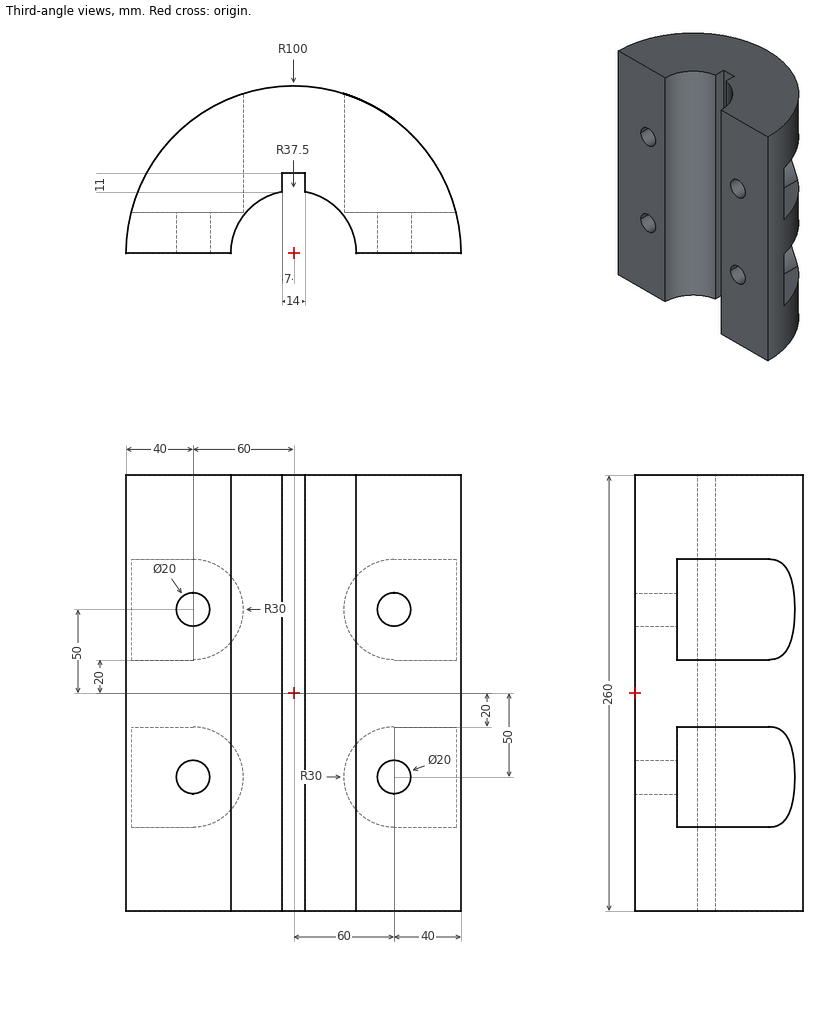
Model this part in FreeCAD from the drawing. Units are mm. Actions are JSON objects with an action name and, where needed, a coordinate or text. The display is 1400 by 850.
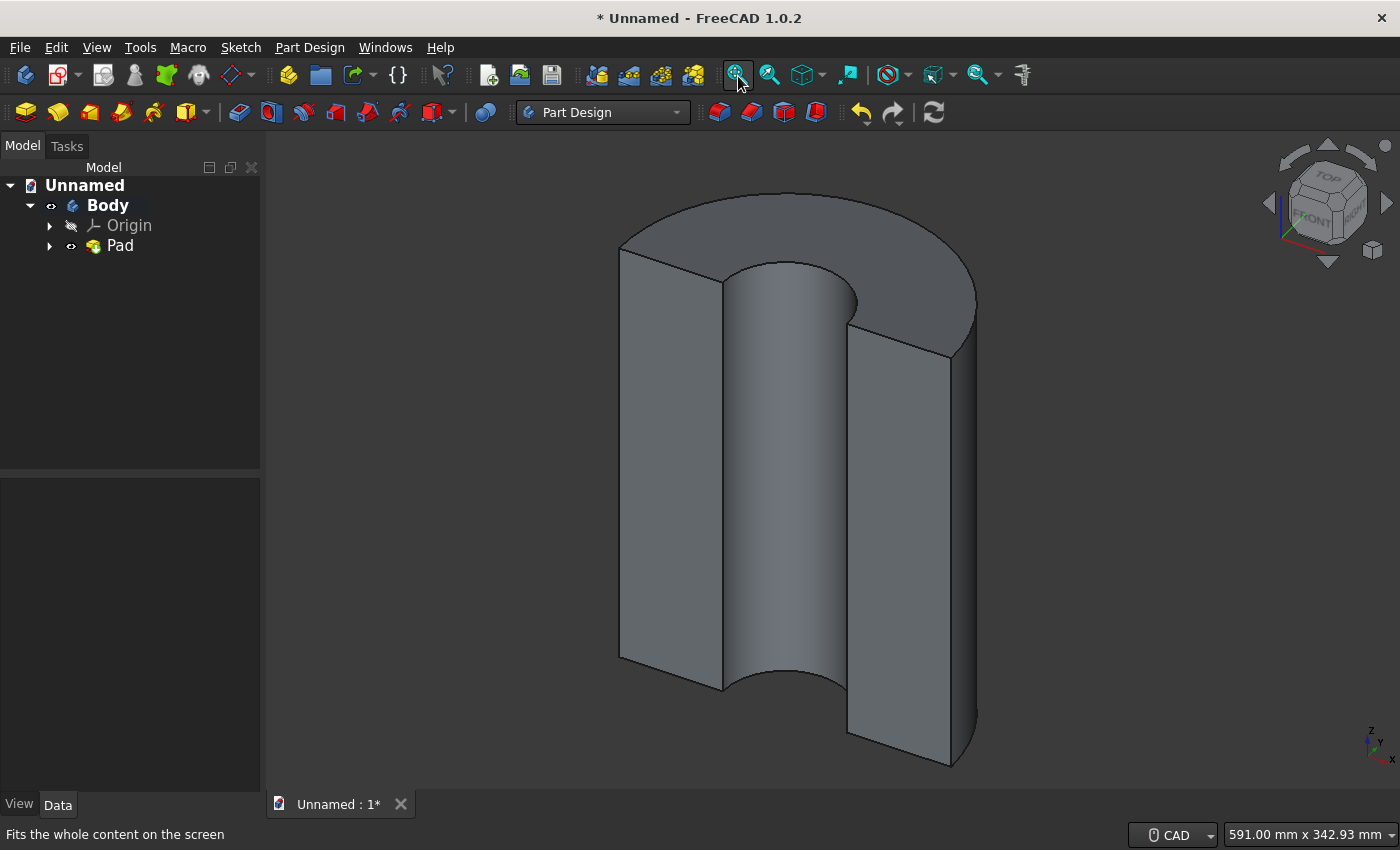
{"action": "left_click", "coordinate": [50, 226]}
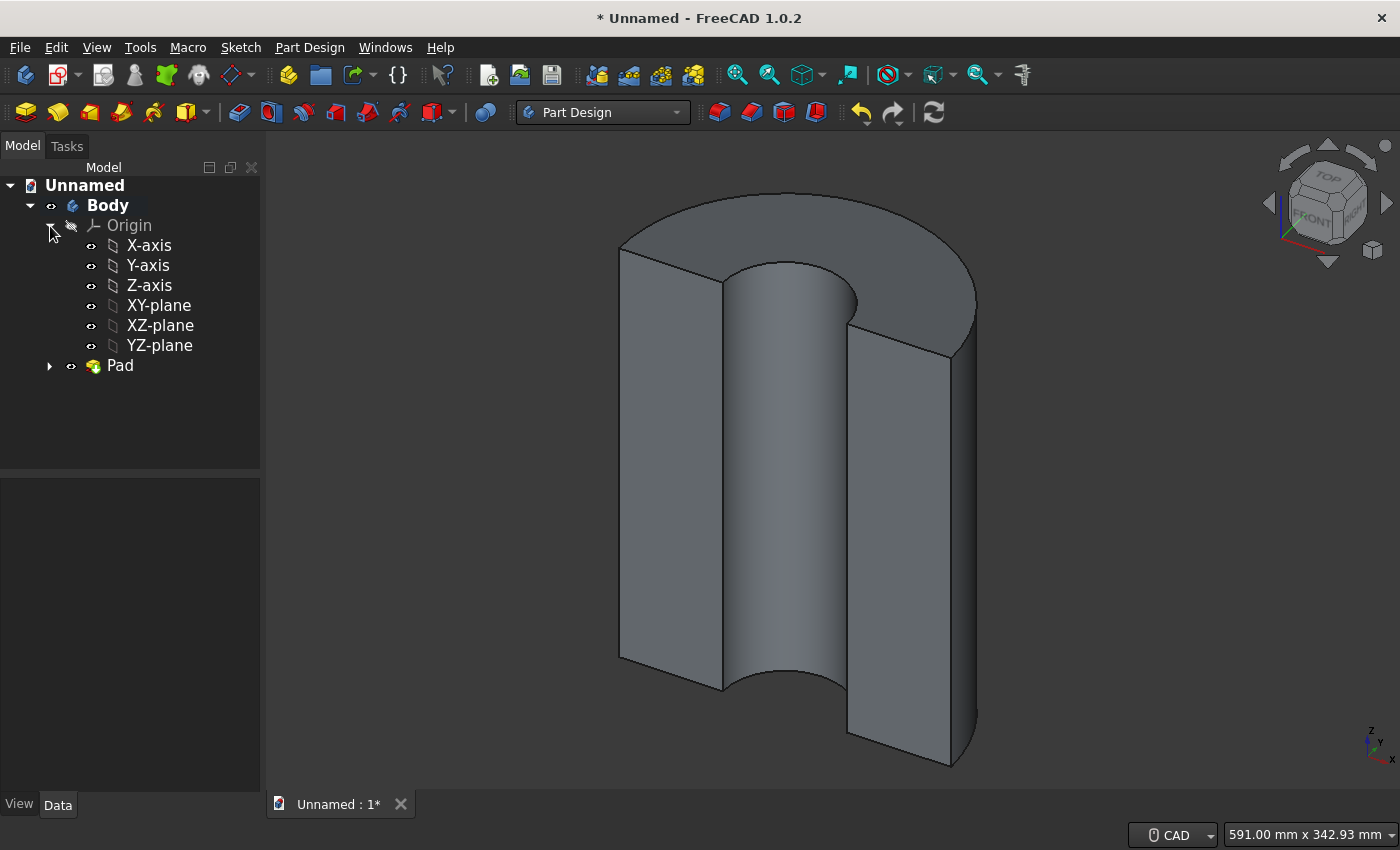
{"action": "left_click", "coordinate": [136, 326]}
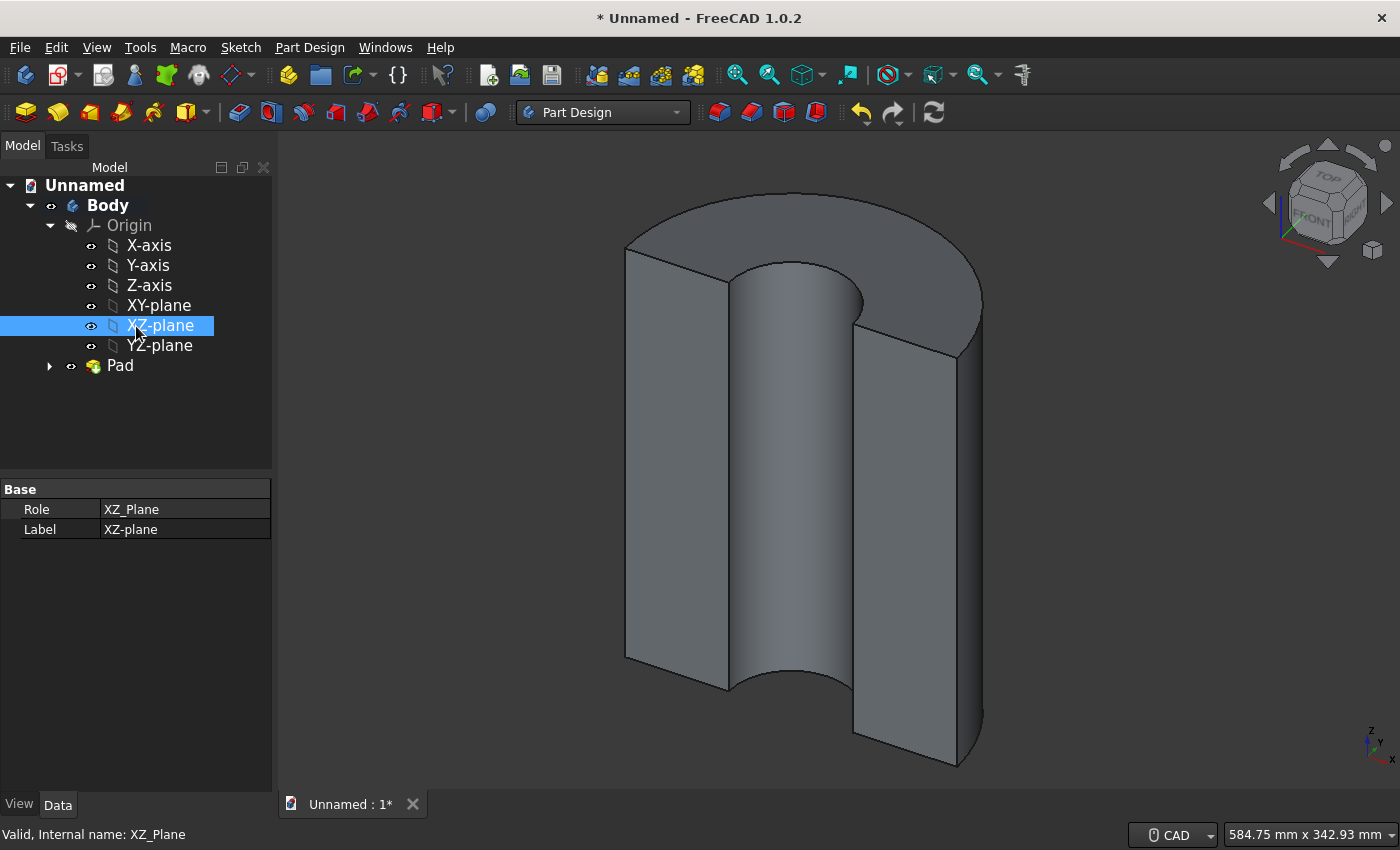
{"action": "left_click", "coordinate": [232, 76]}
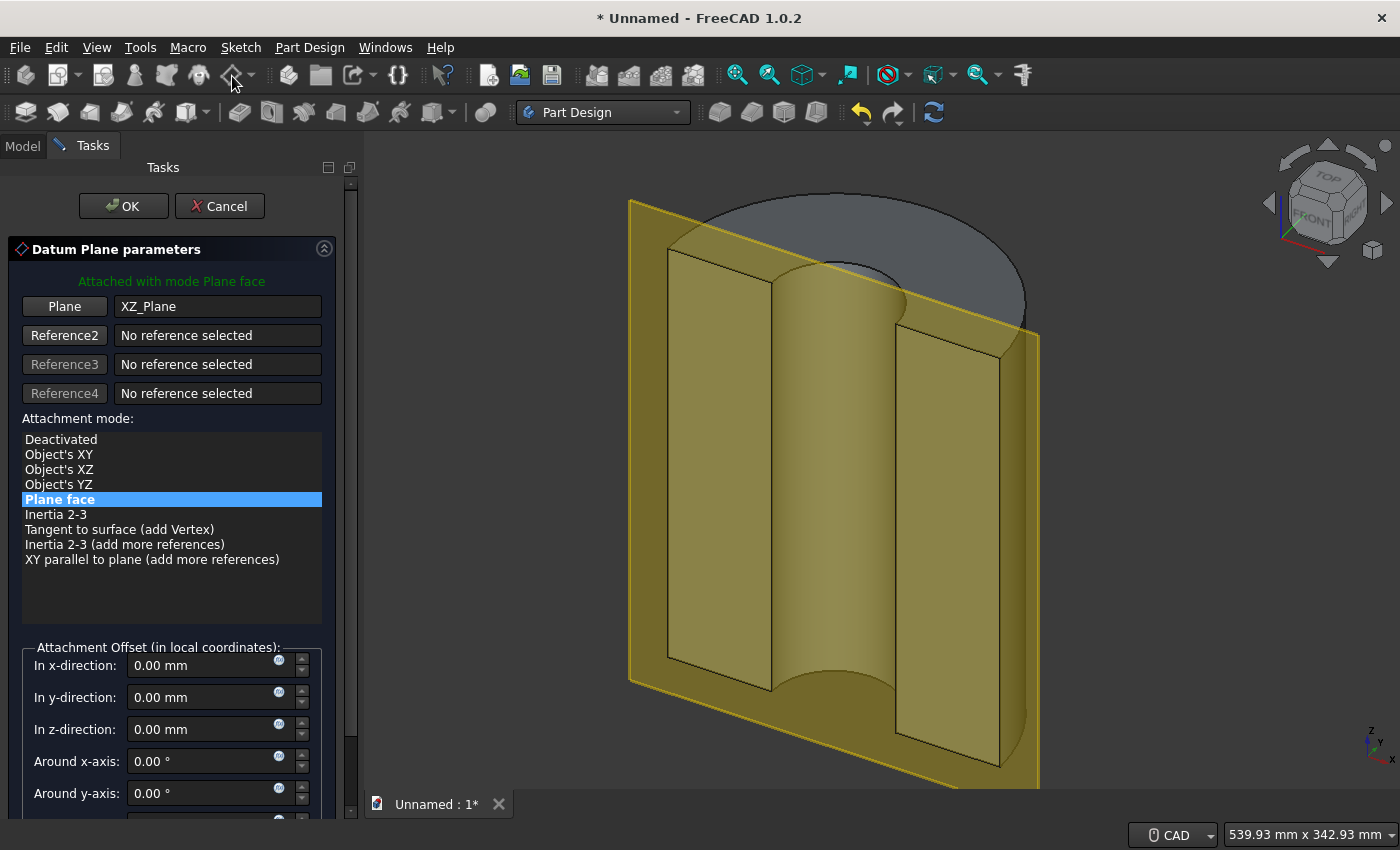
{"action": "triple_click", "coordinate": [210, 729]}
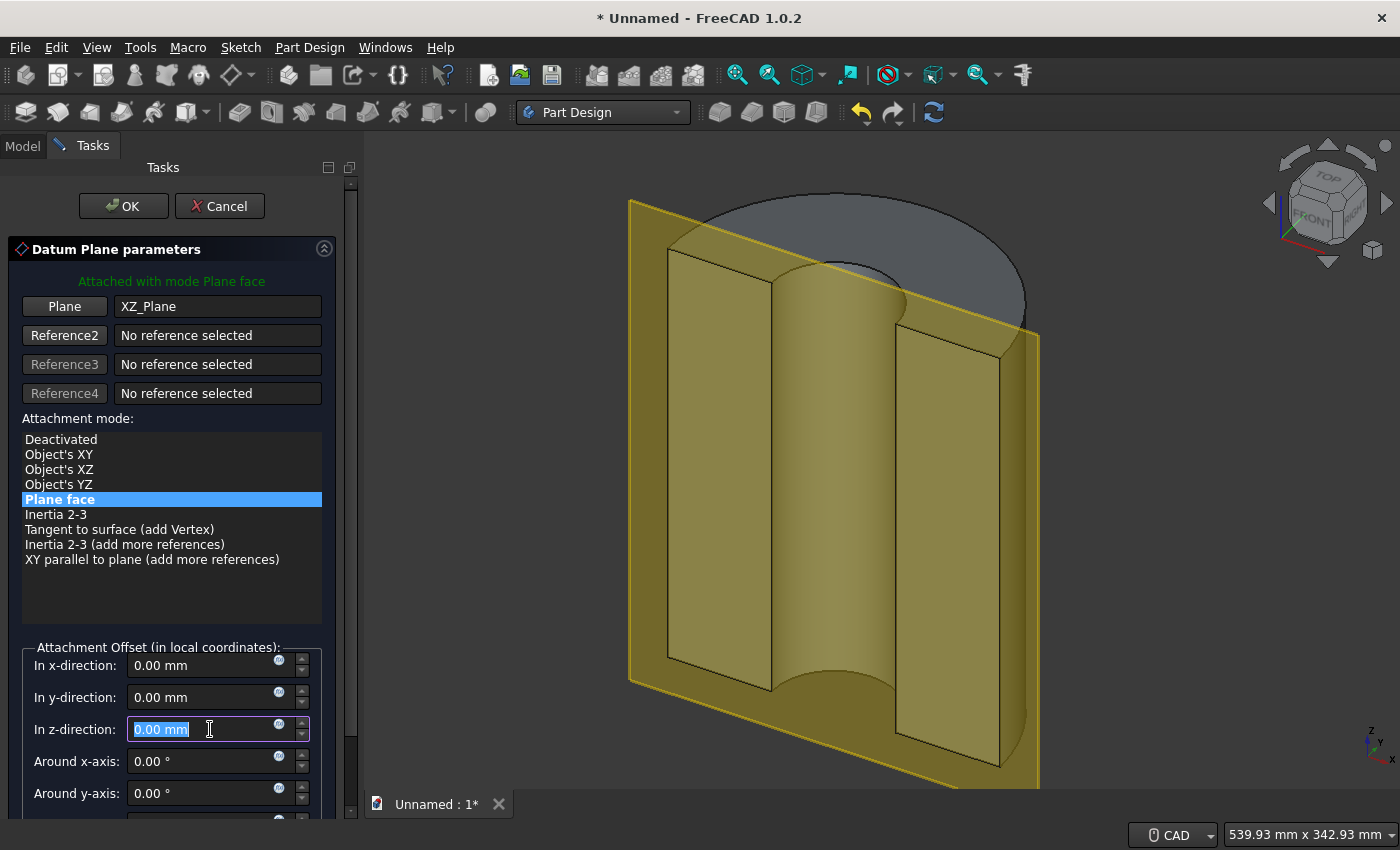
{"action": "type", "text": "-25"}
{"action": "key", "text": "Tab"}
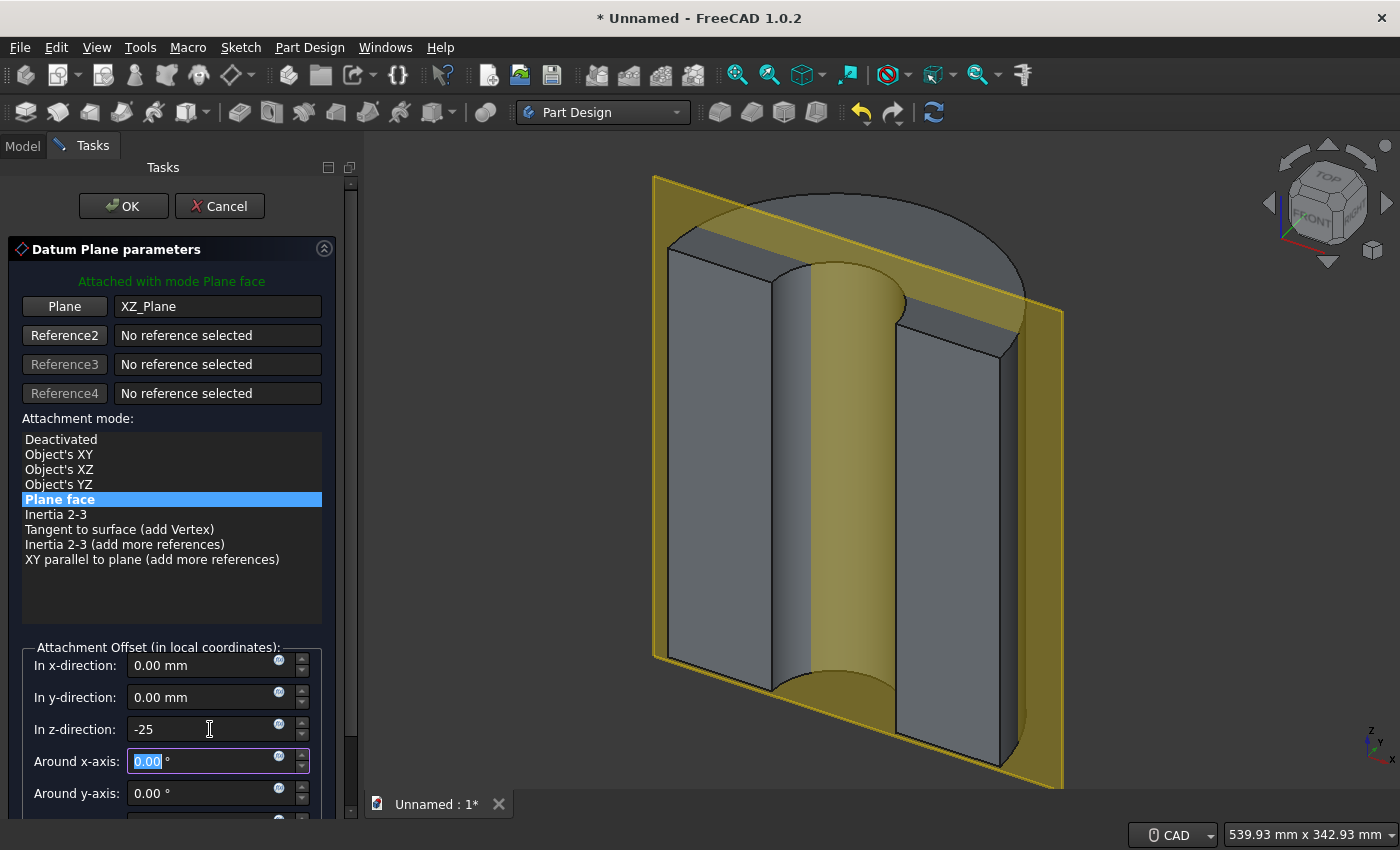
{"action": "left_click", "coordinate": [124, 206]}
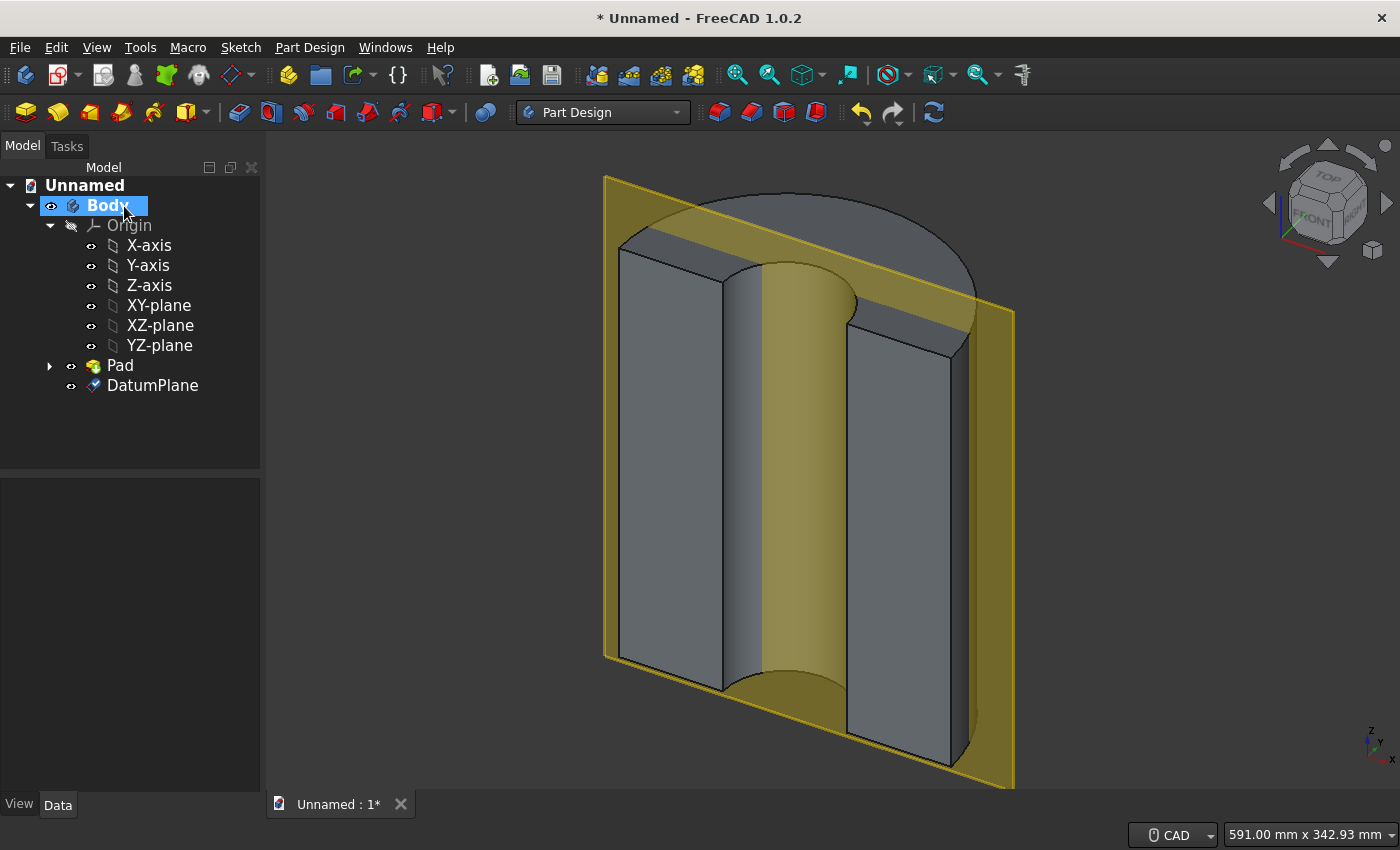
{"action": "left_click", "coordinate": [116, 386]}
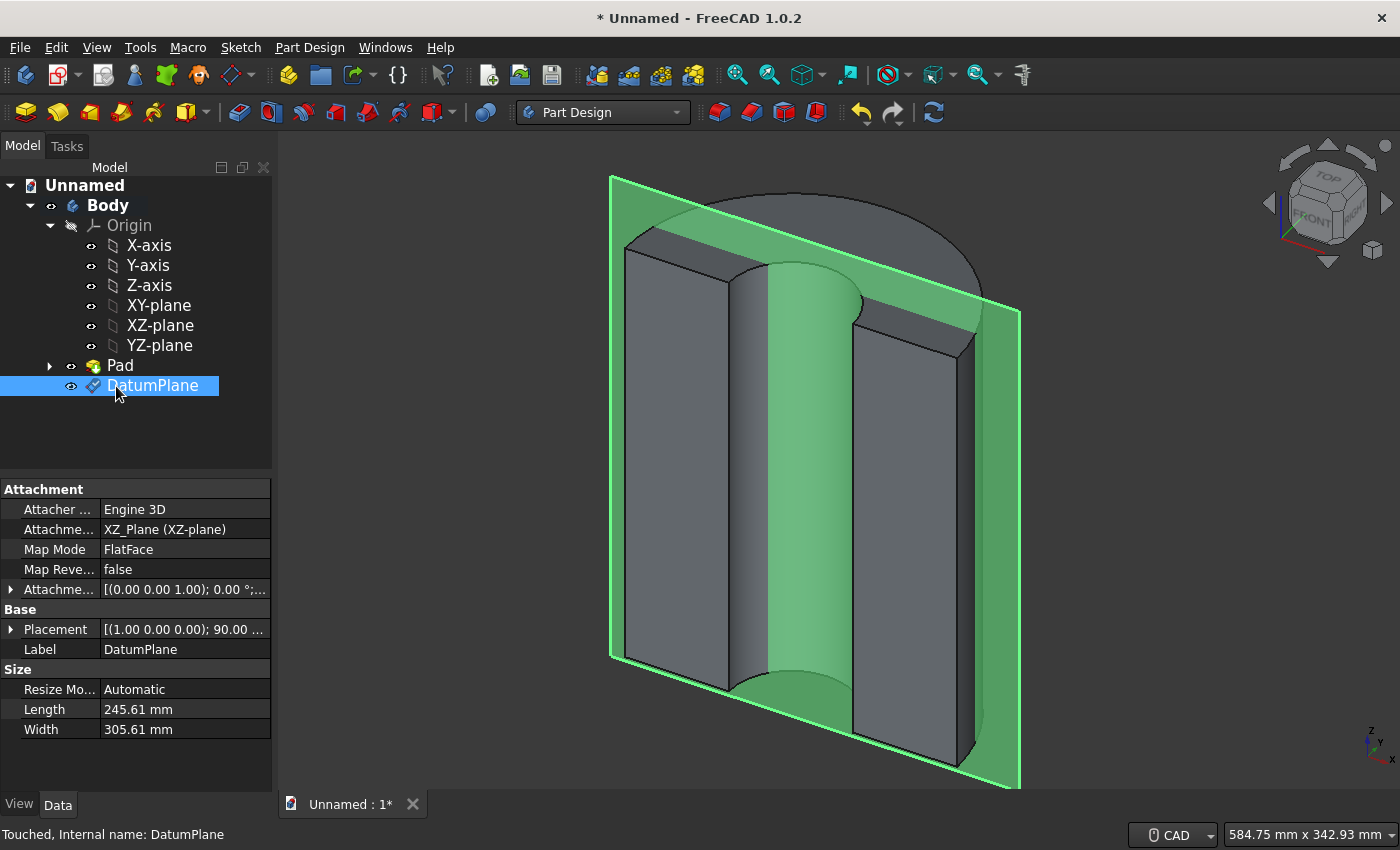
{"action": "left_click", "coordinate": [58, 76]}